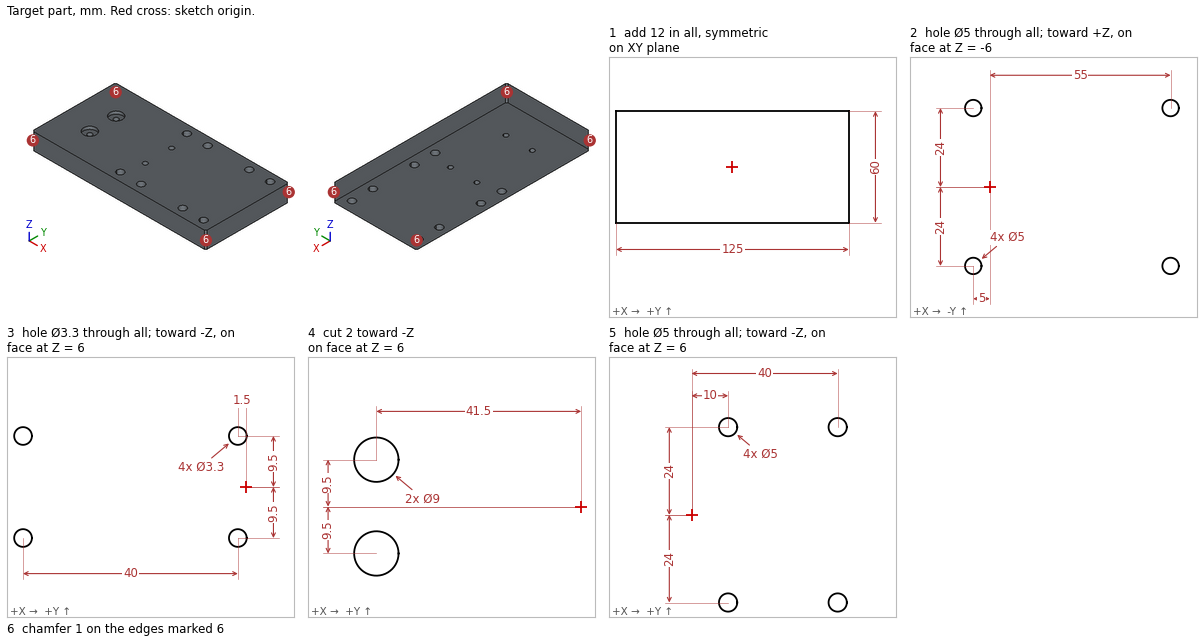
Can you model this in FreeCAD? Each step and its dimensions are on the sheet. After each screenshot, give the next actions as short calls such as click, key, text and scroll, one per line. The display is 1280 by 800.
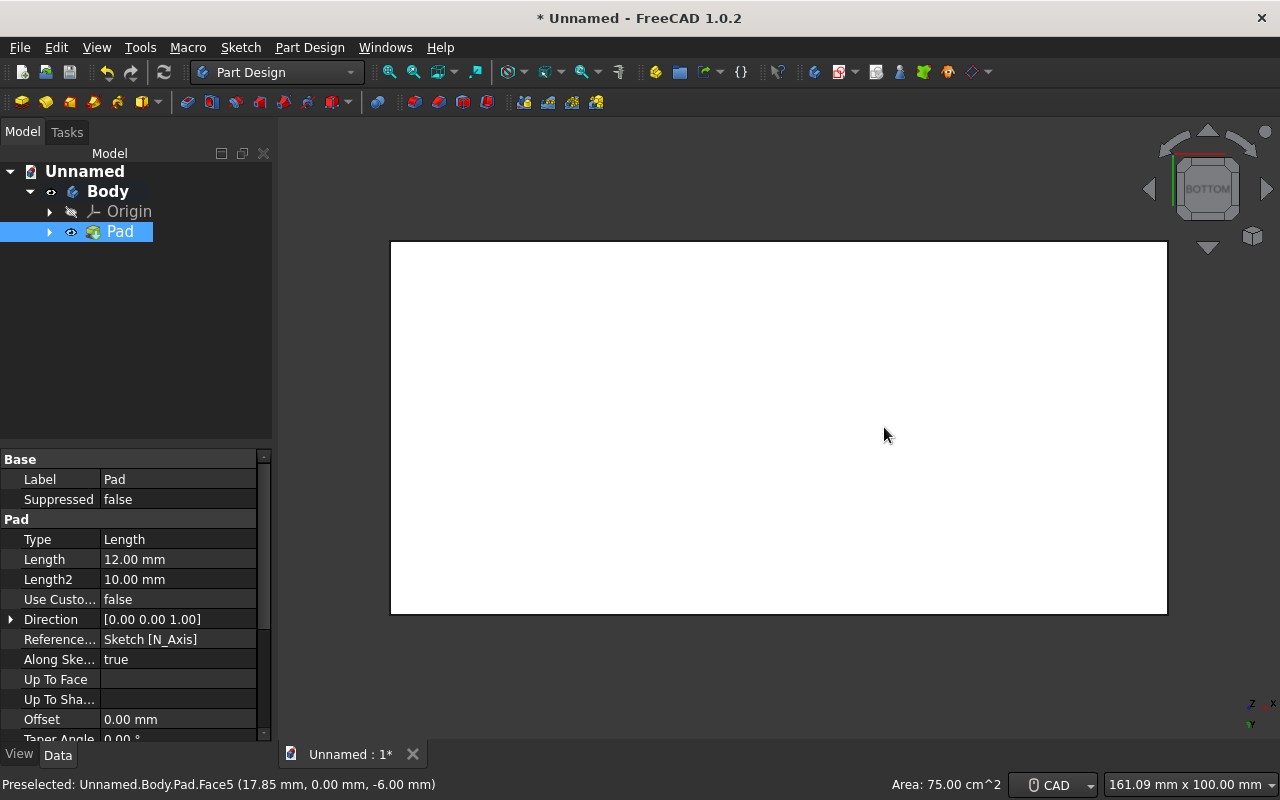
click(840, 72)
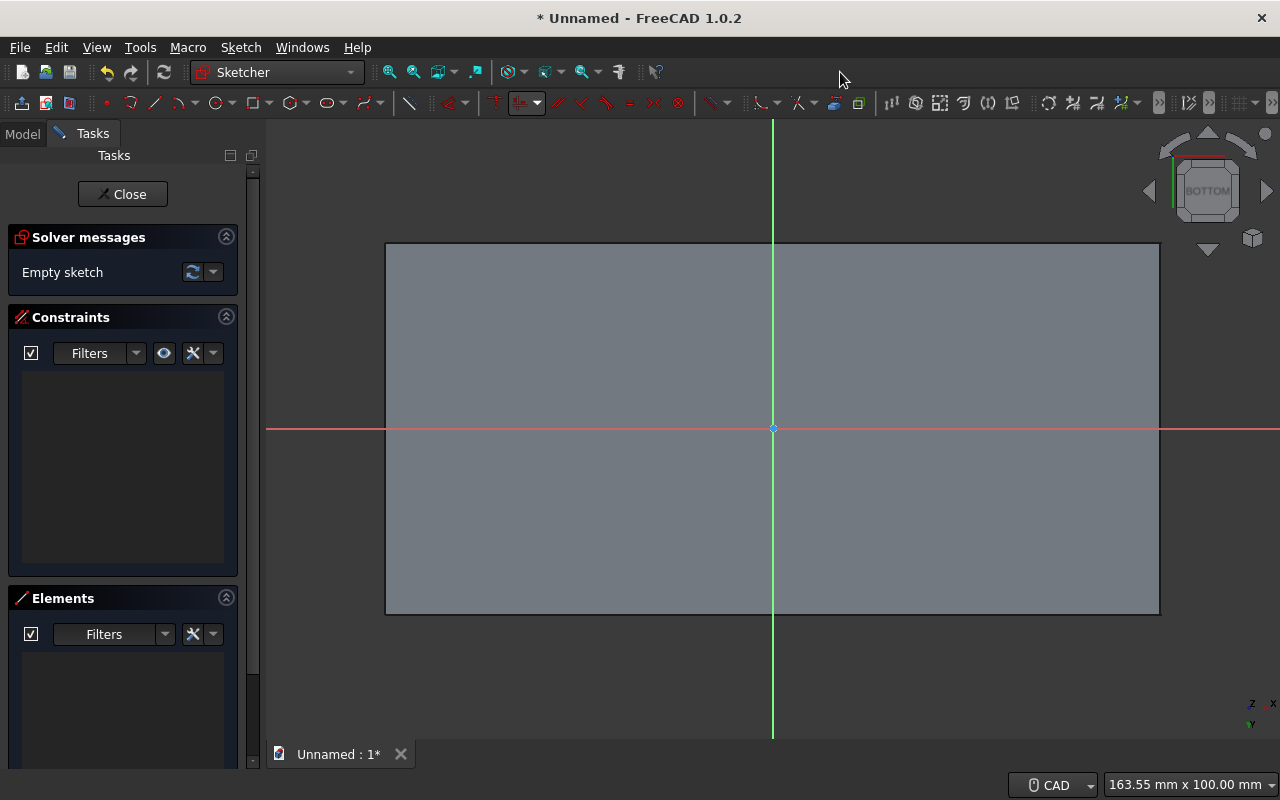
scroll(294, 429, down, 1)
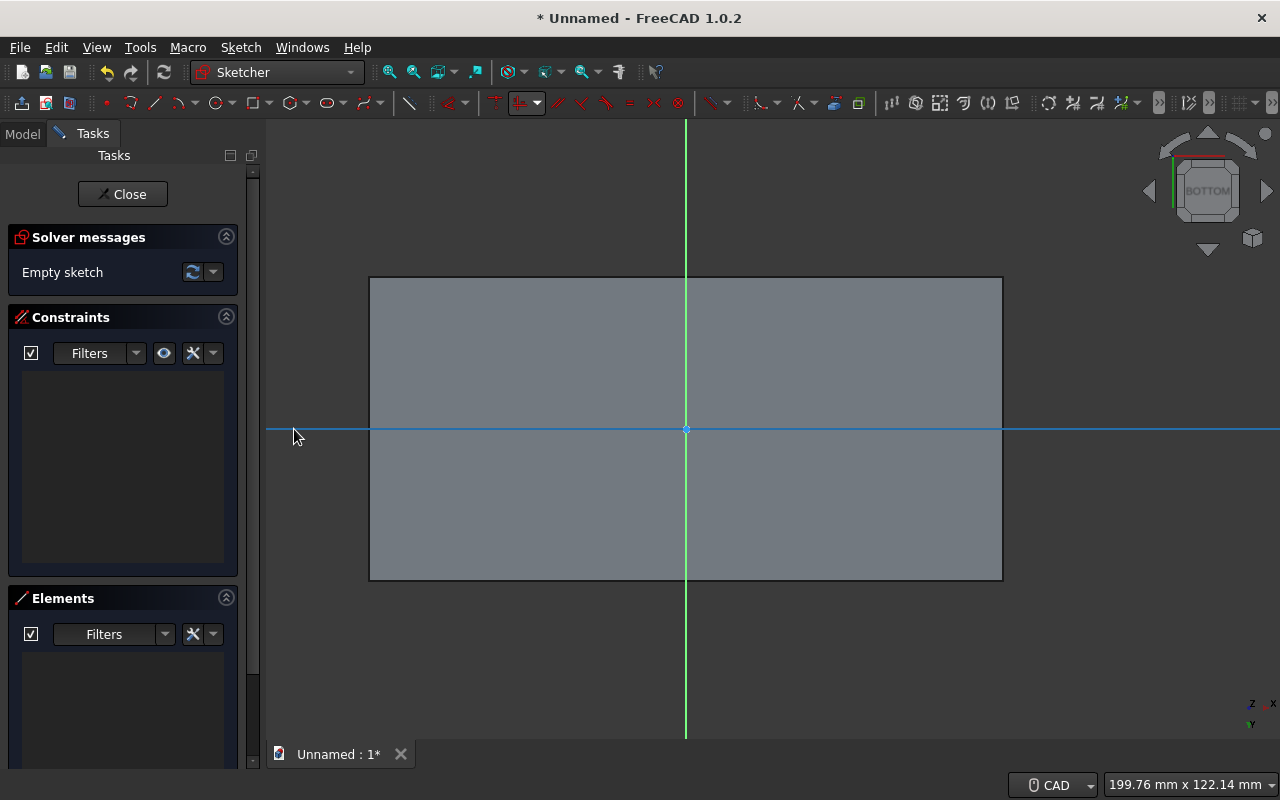
scroll(1034, 429, up, 2)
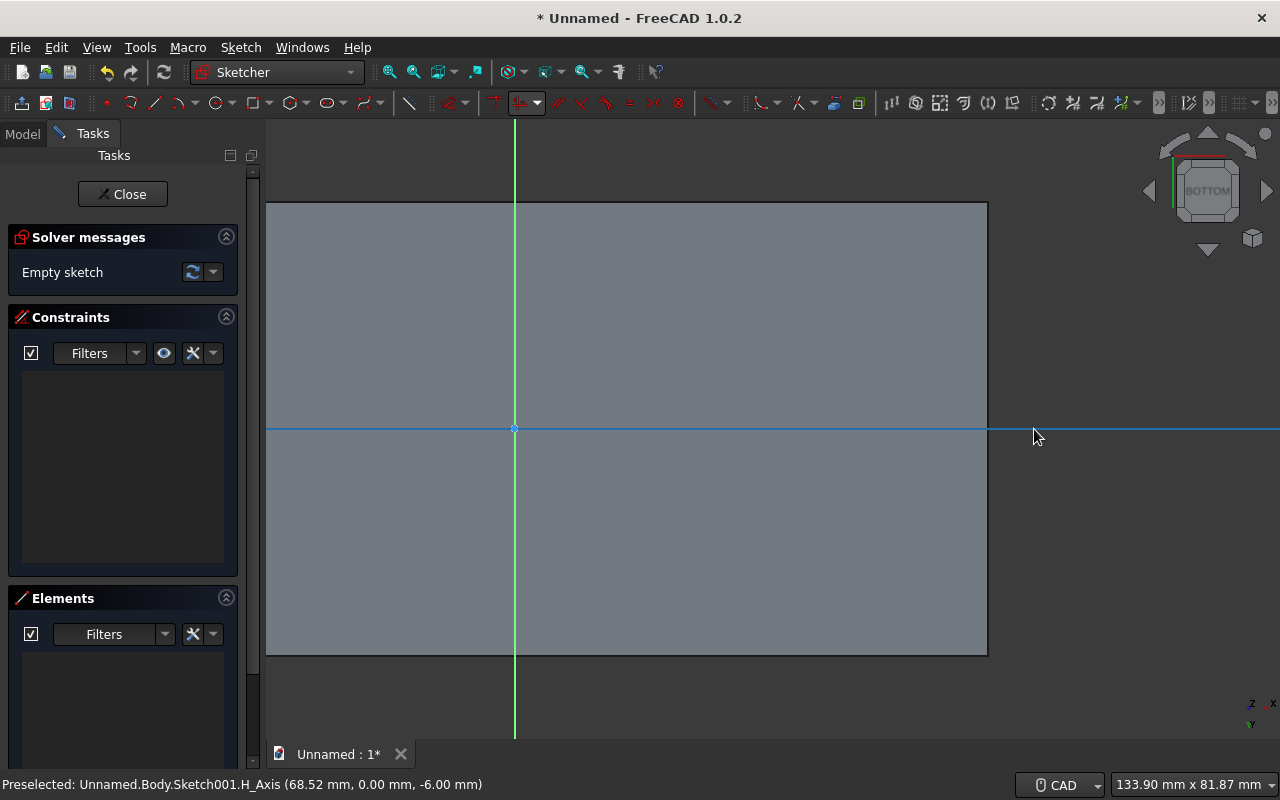
key(g)
key(c)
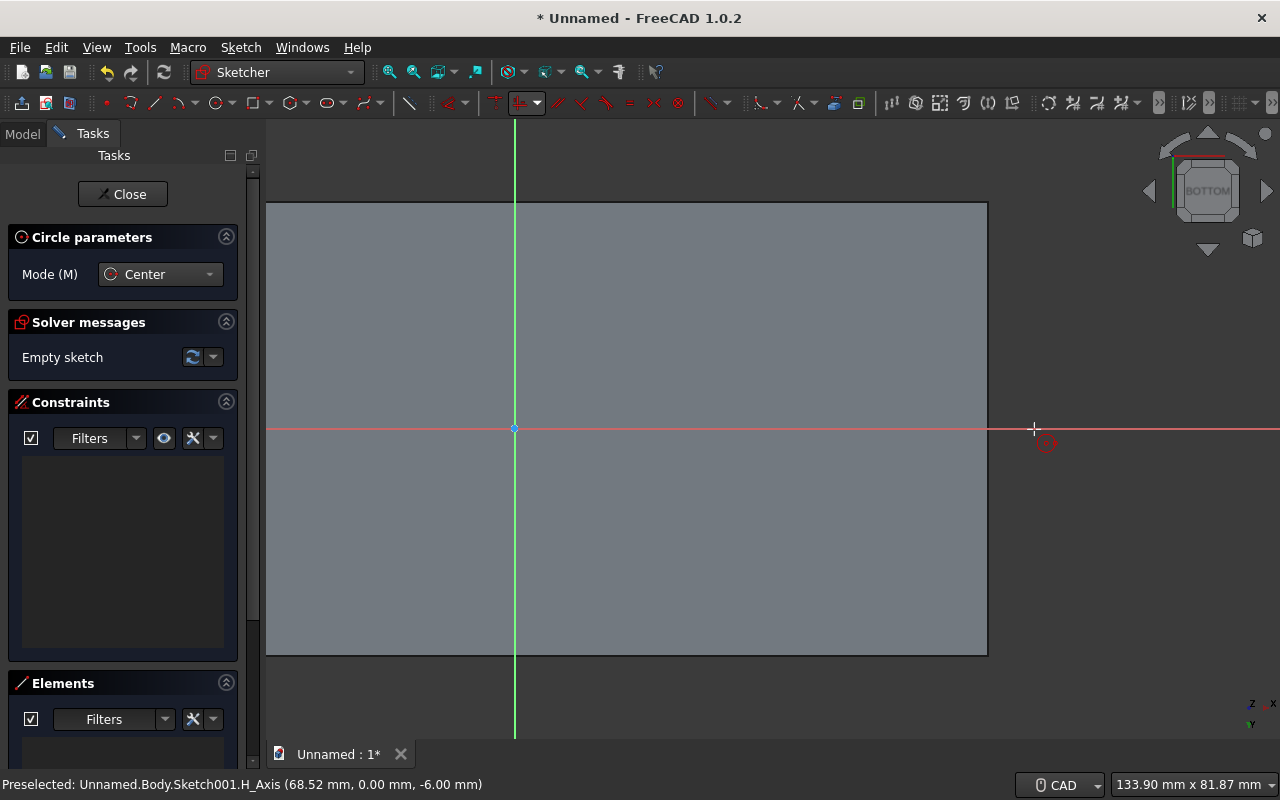
click(477, 611)
click(490, 597)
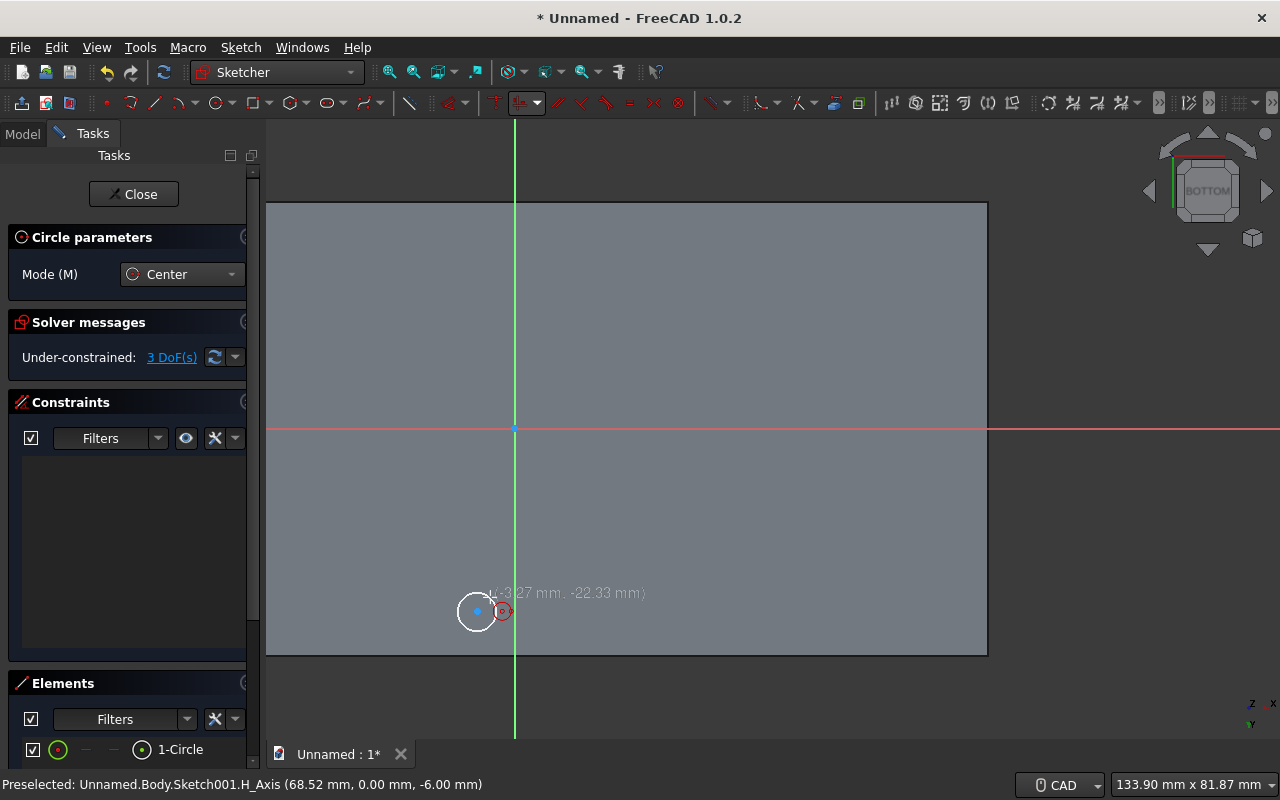
click(477, 247)
click(490, 234)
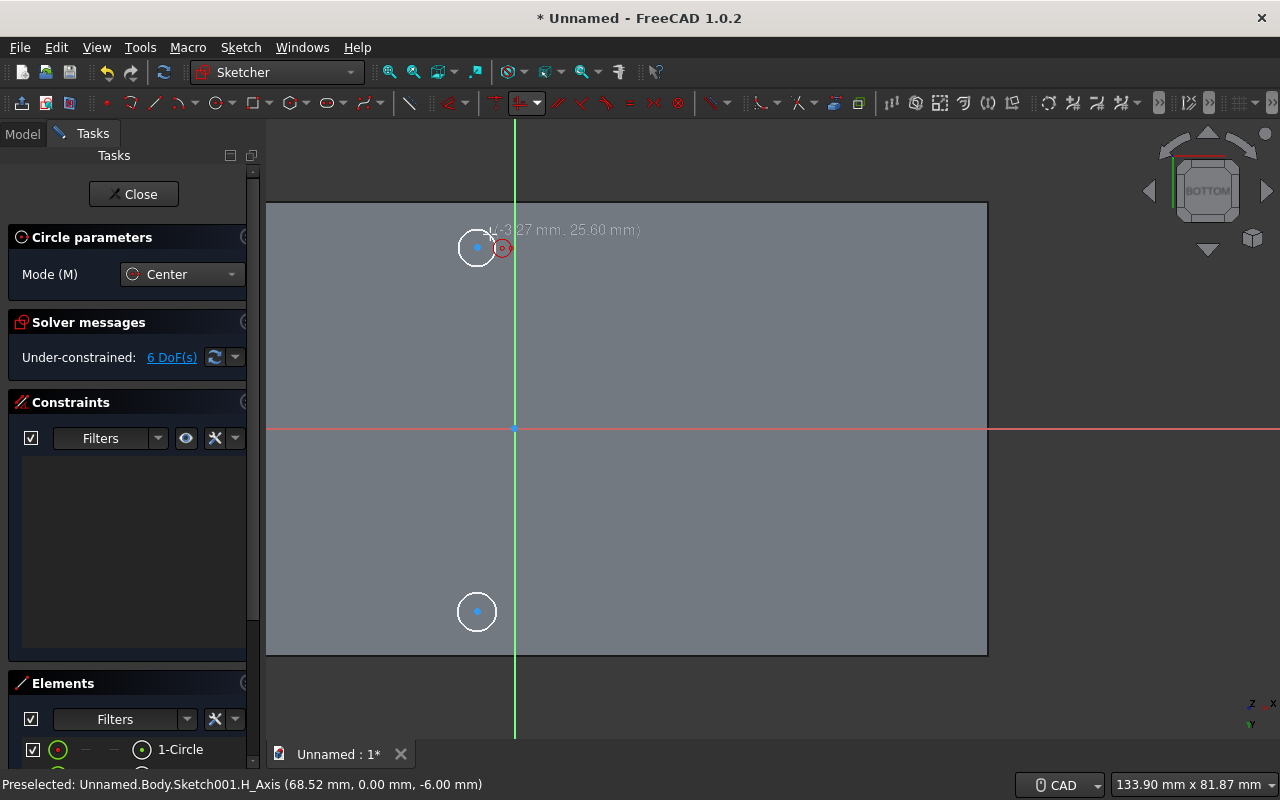
click(931, 247)
click(945, 234)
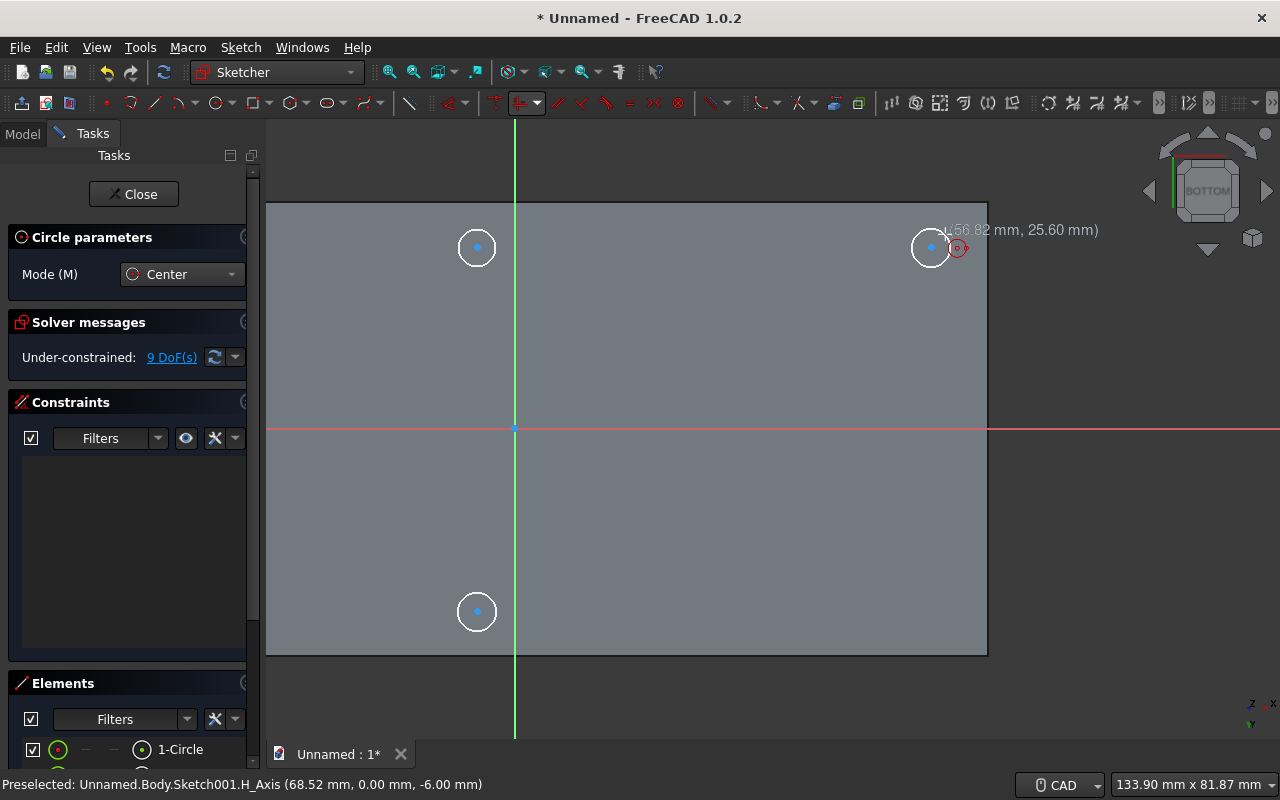
click(931, 611)
click(945, 597)
key(Escape)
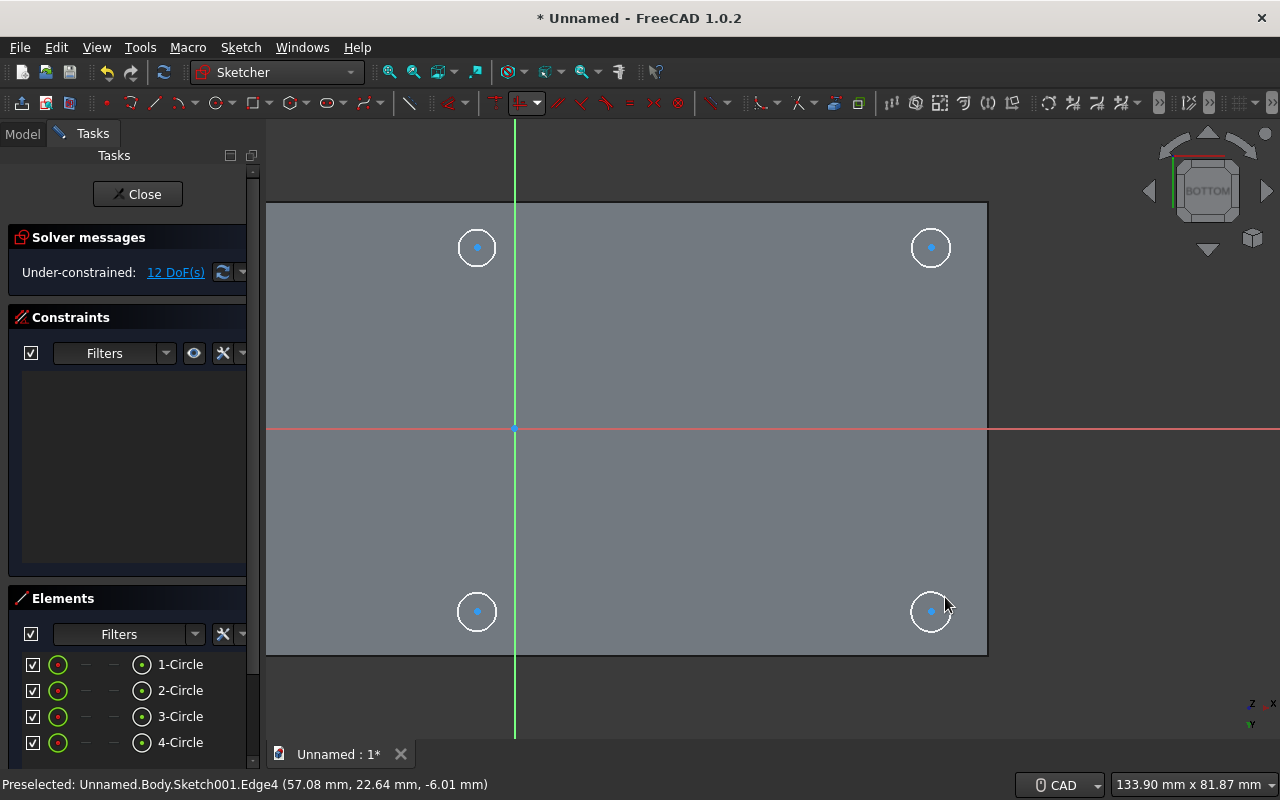
click(490, 598)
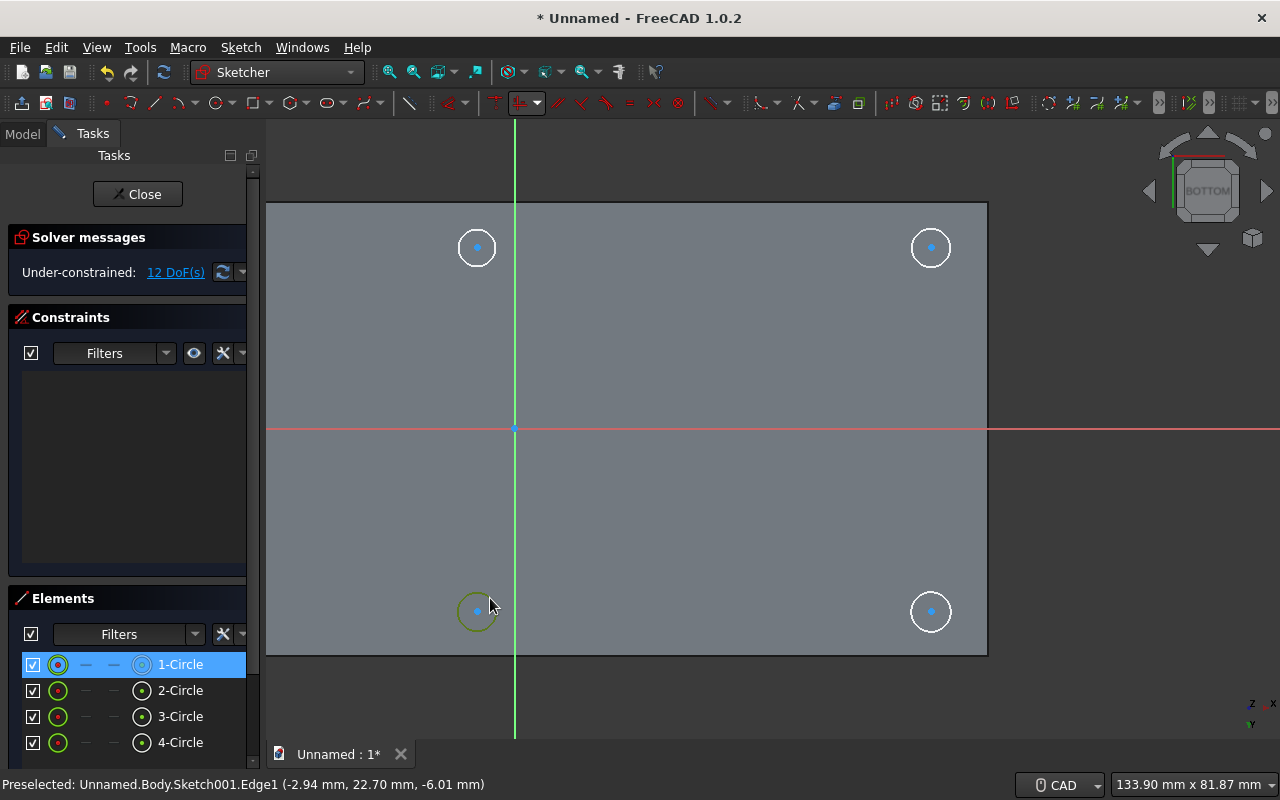
click(490, 235)